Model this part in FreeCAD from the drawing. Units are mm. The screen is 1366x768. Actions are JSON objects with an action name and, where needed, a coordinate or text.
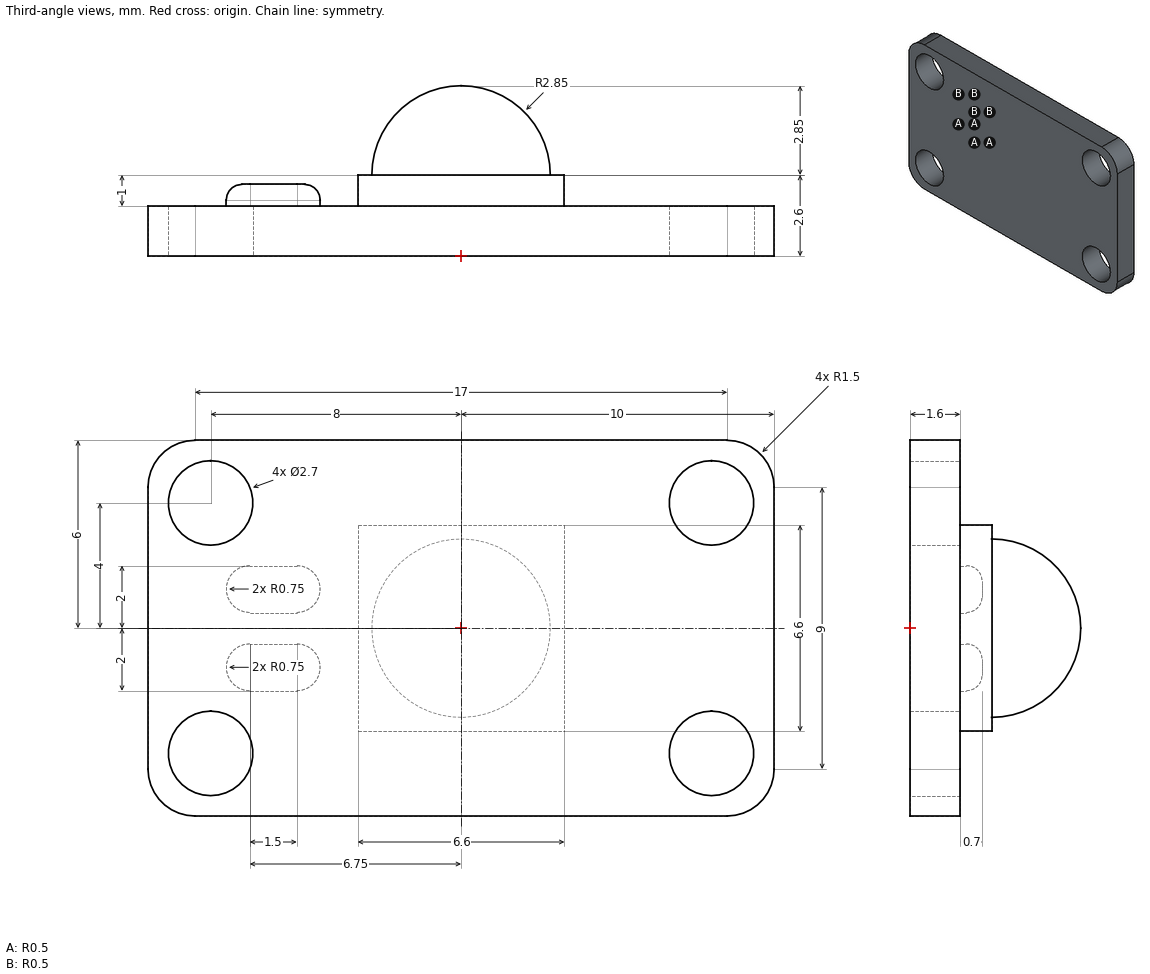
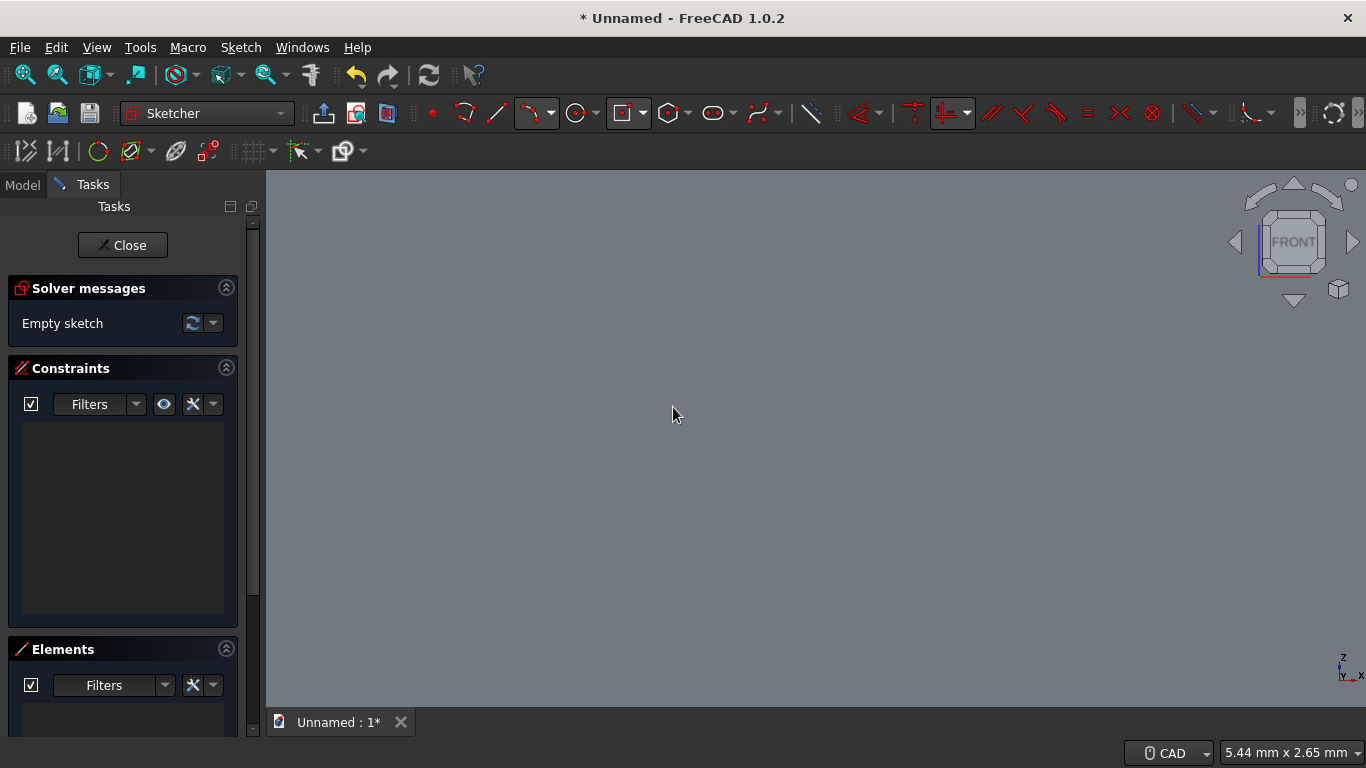
{"action": "left_click", "coordinate": [714, 114]}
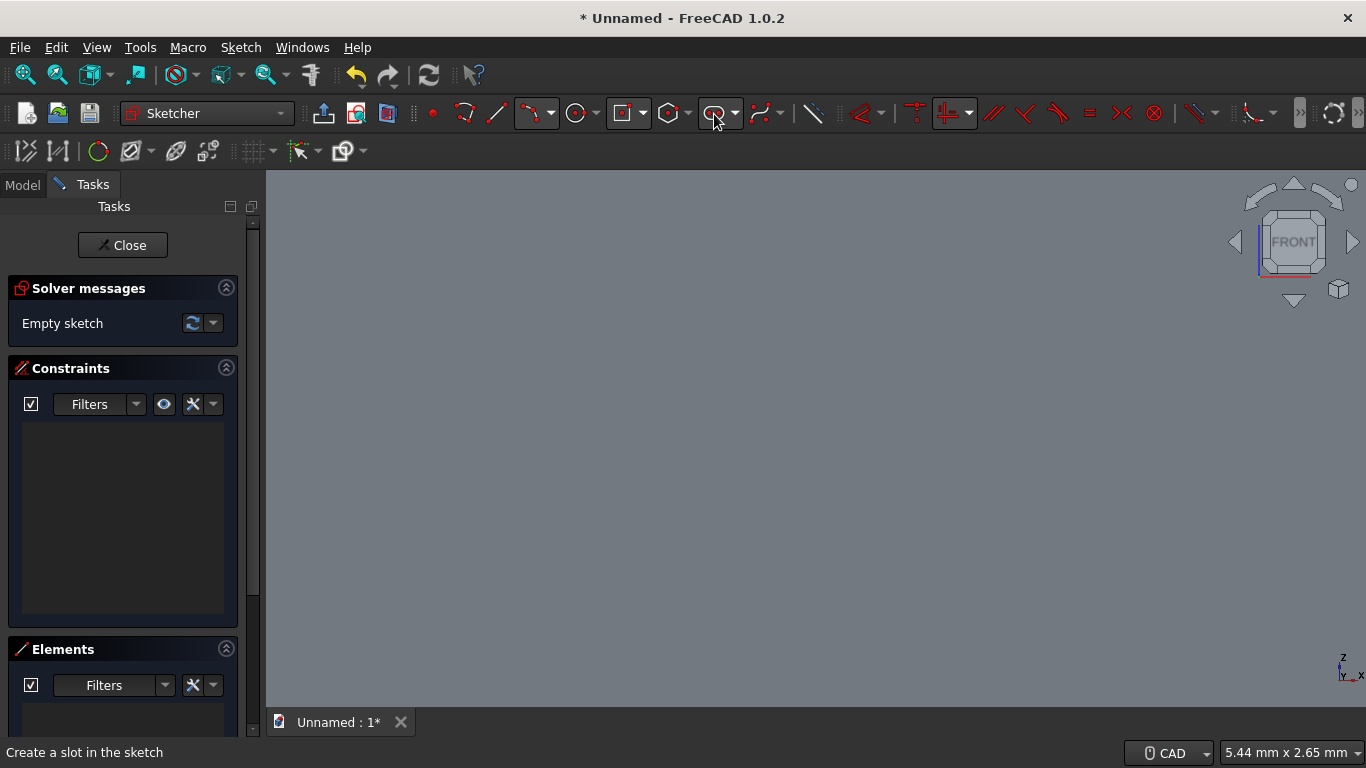
{"action": "left_click", "coordinate": [595, 435]}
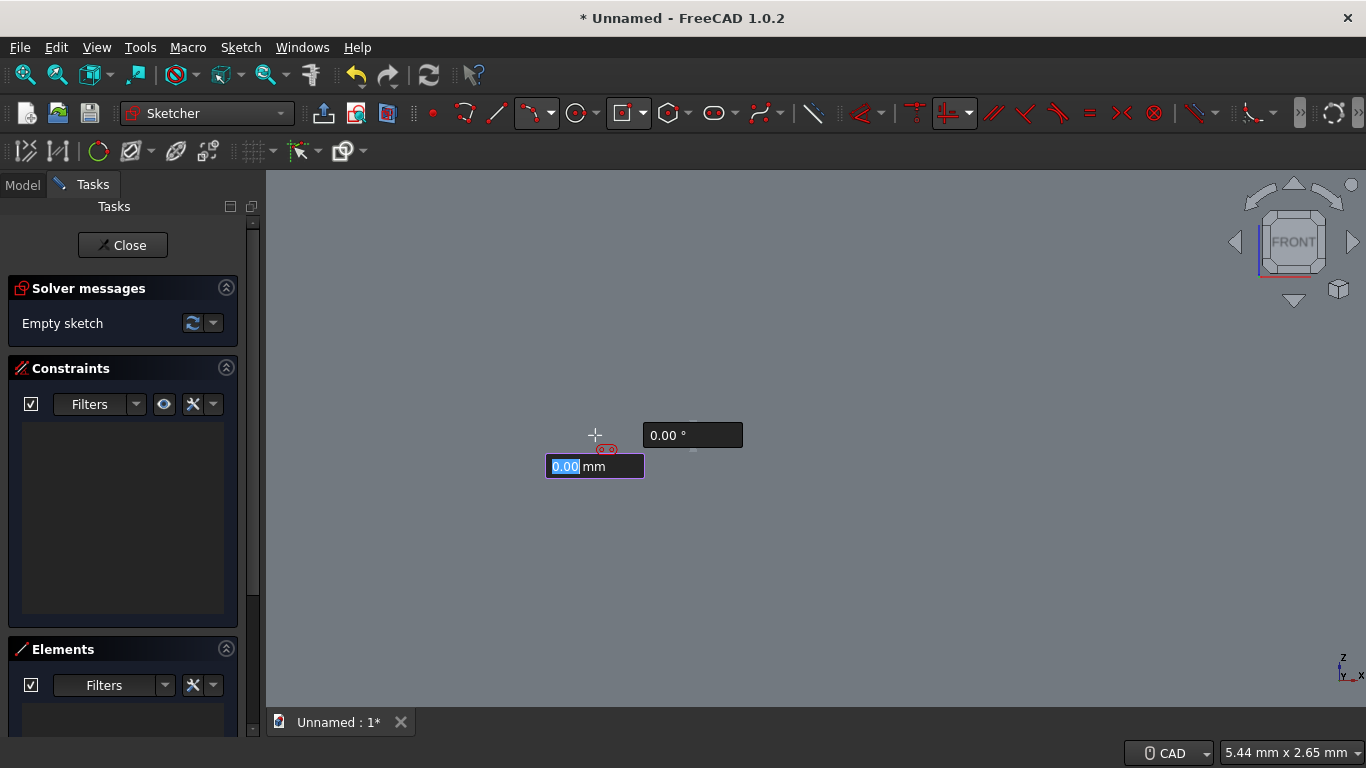
{"action": "left_click", "coordinate": [898, 435]}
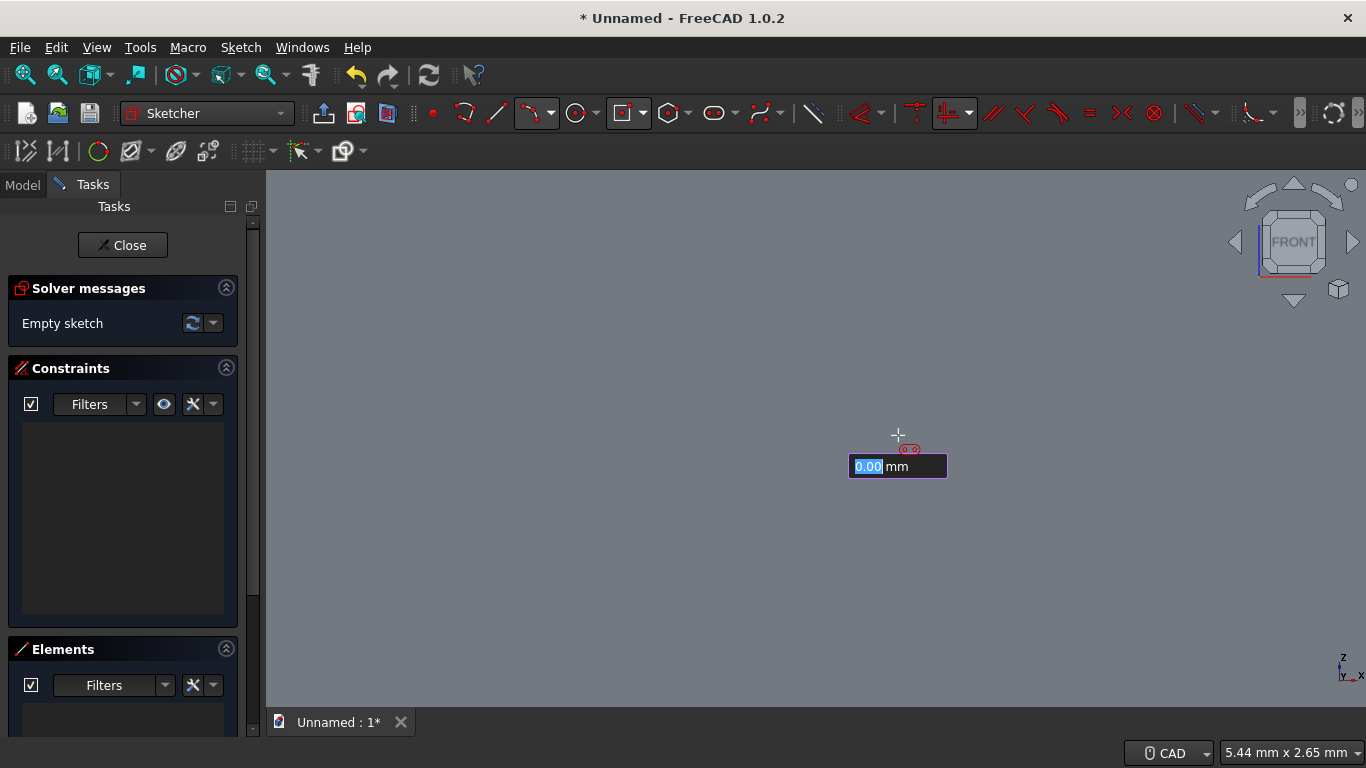
{"action": "left_click", "coordinate": [747, 587]}
{"action": "key", "text": "Escape"}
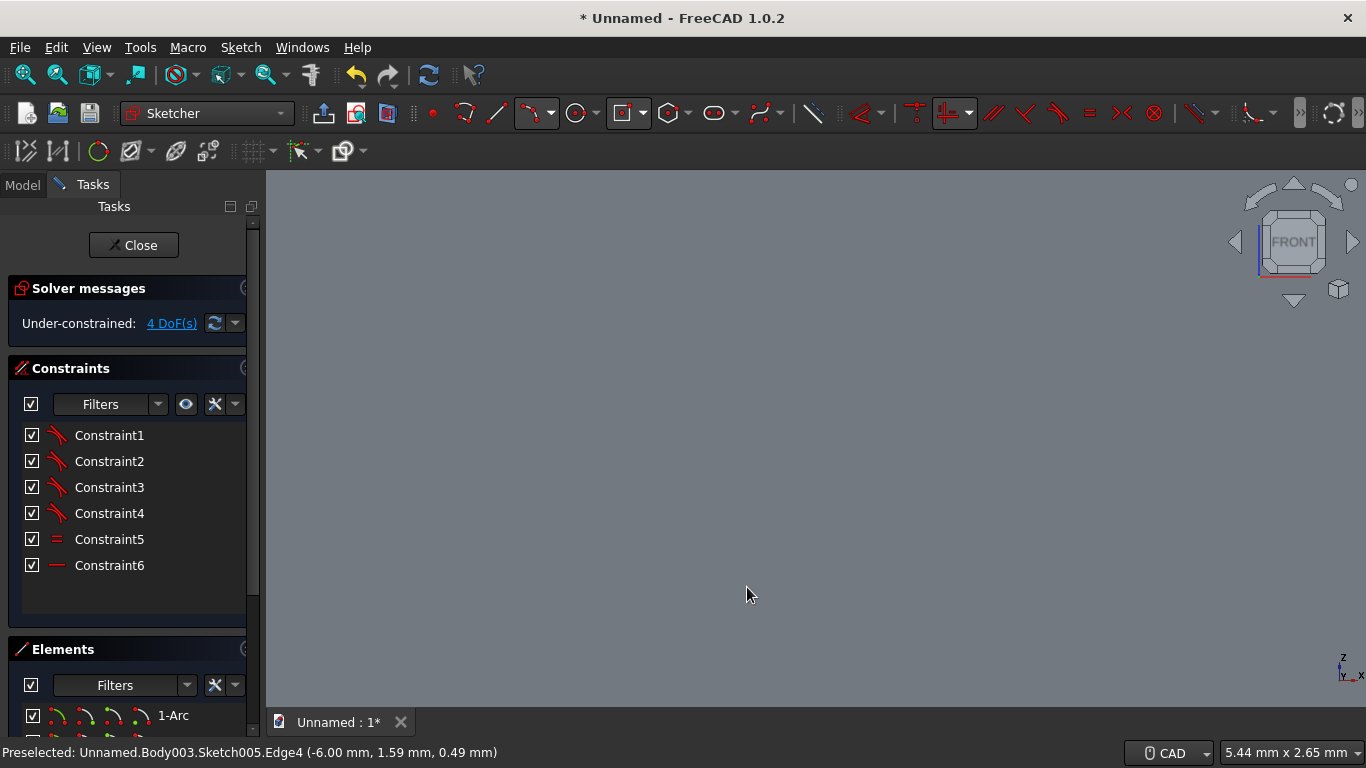
{"action": "left_click", "coordinate": [860, 114]}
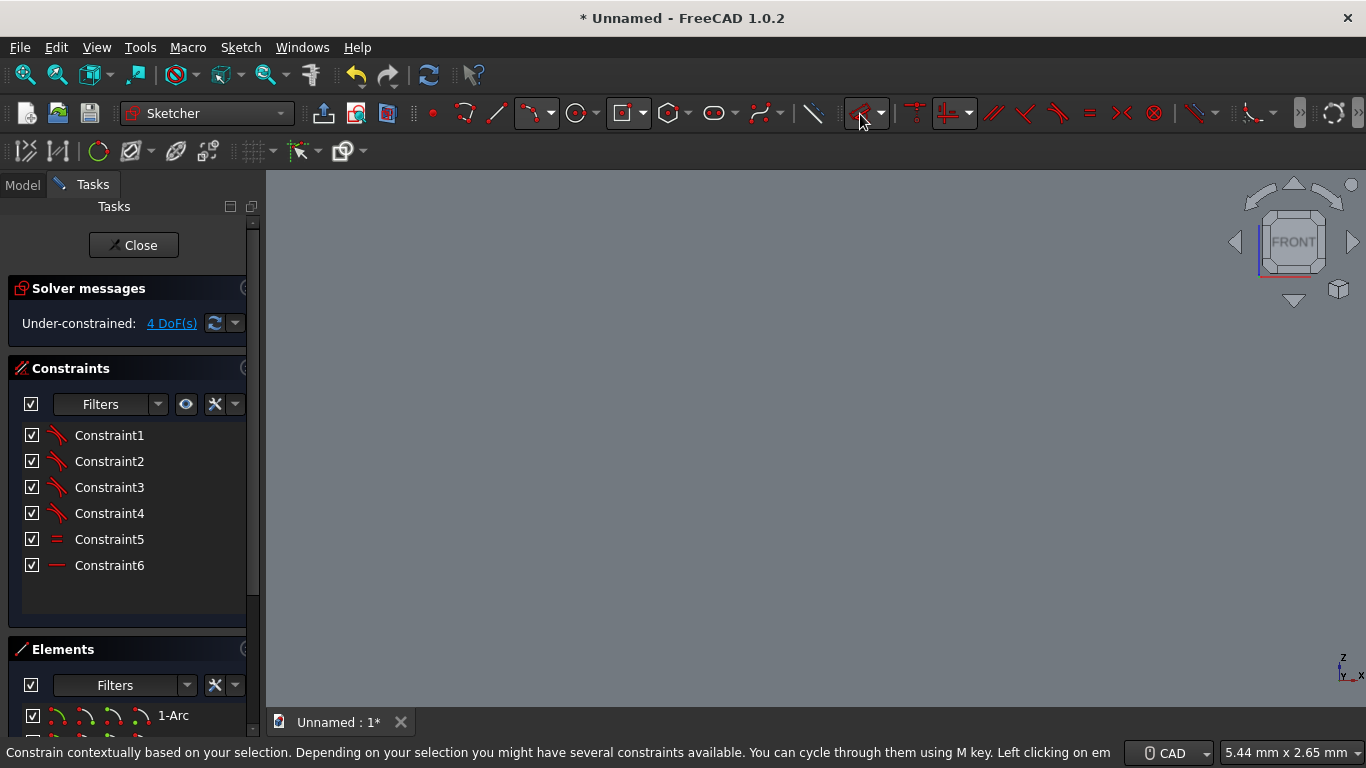
{"action": "left_click", "coordinate": [472, 347]}
{"action": "left_click", "coordinate": [446, 328]}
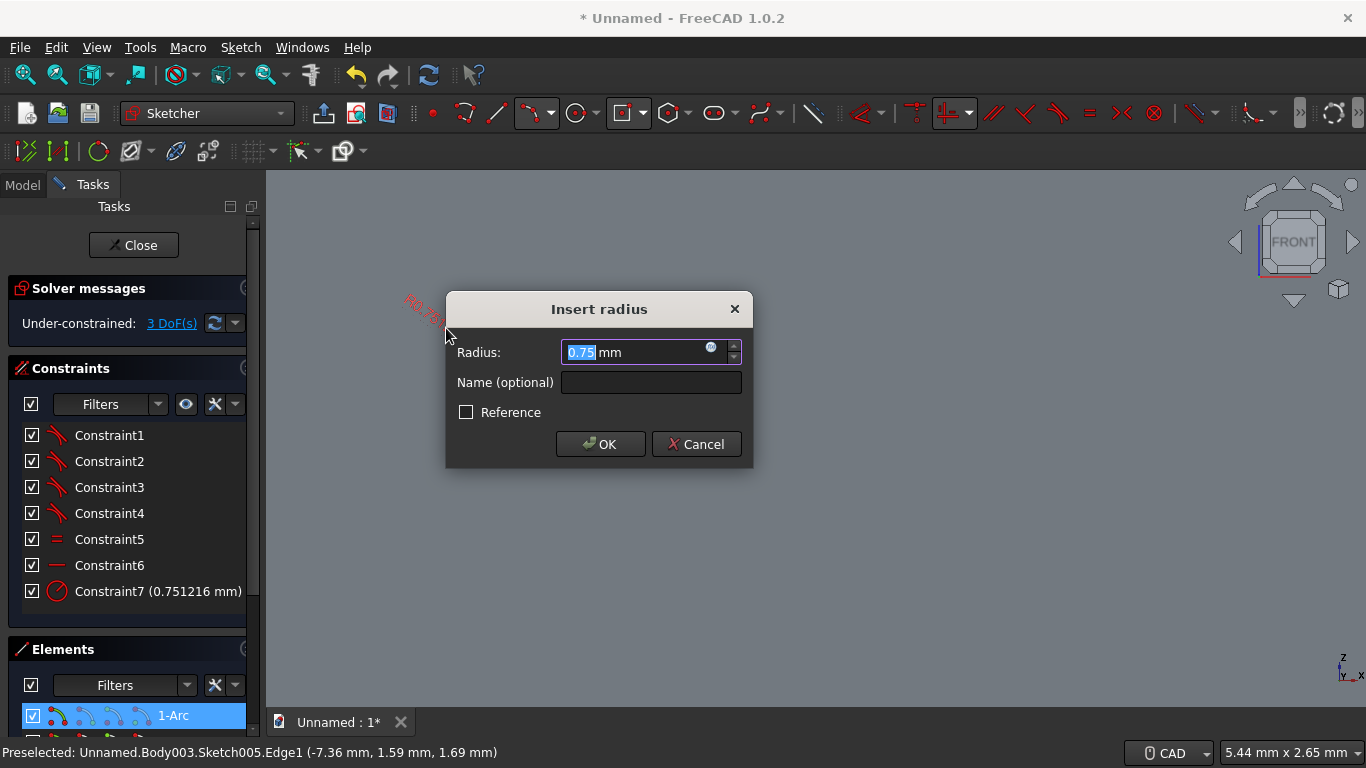
{"action": "type", "text": "0.75"}
{"action": "key", "text": "Return"}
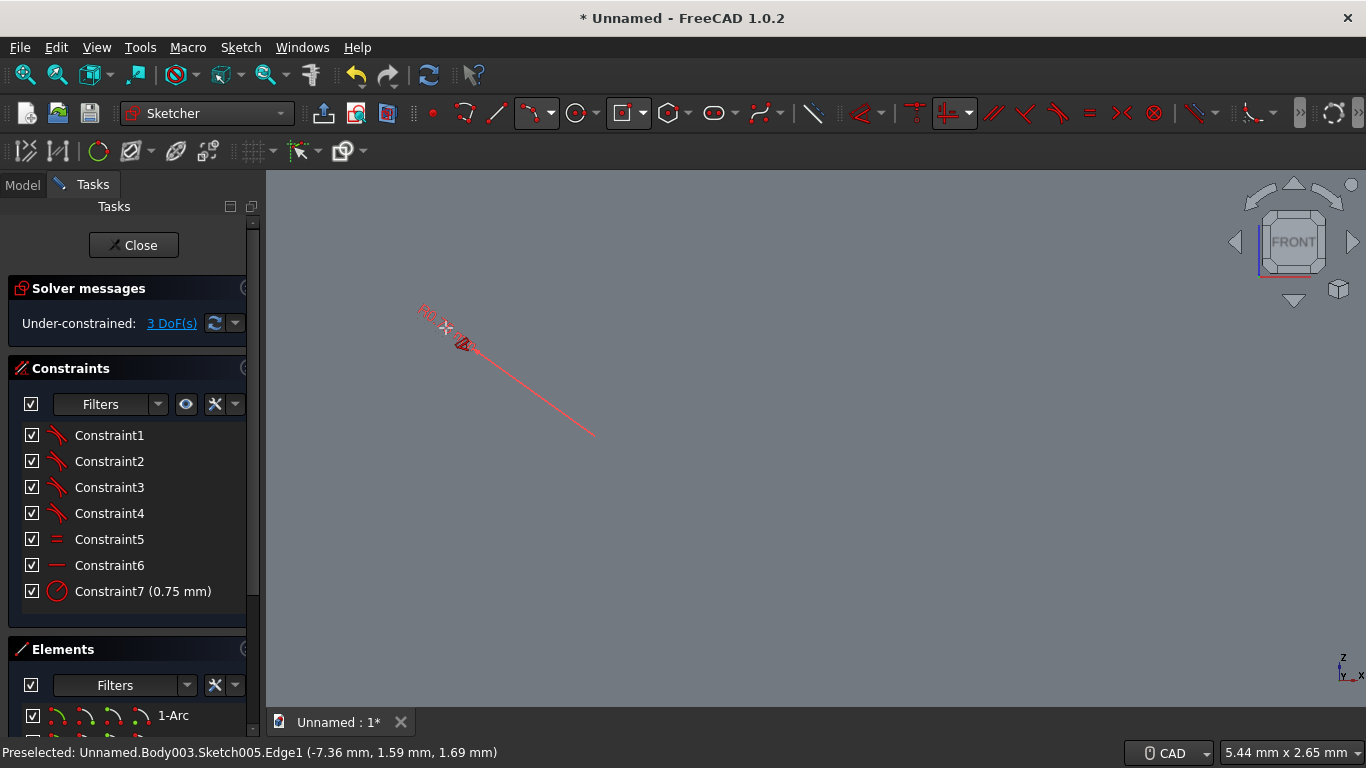
{"action": "left_click", "coordinate": [595, 284]}
{"action": "left_click", "coordinate": [561, 482]}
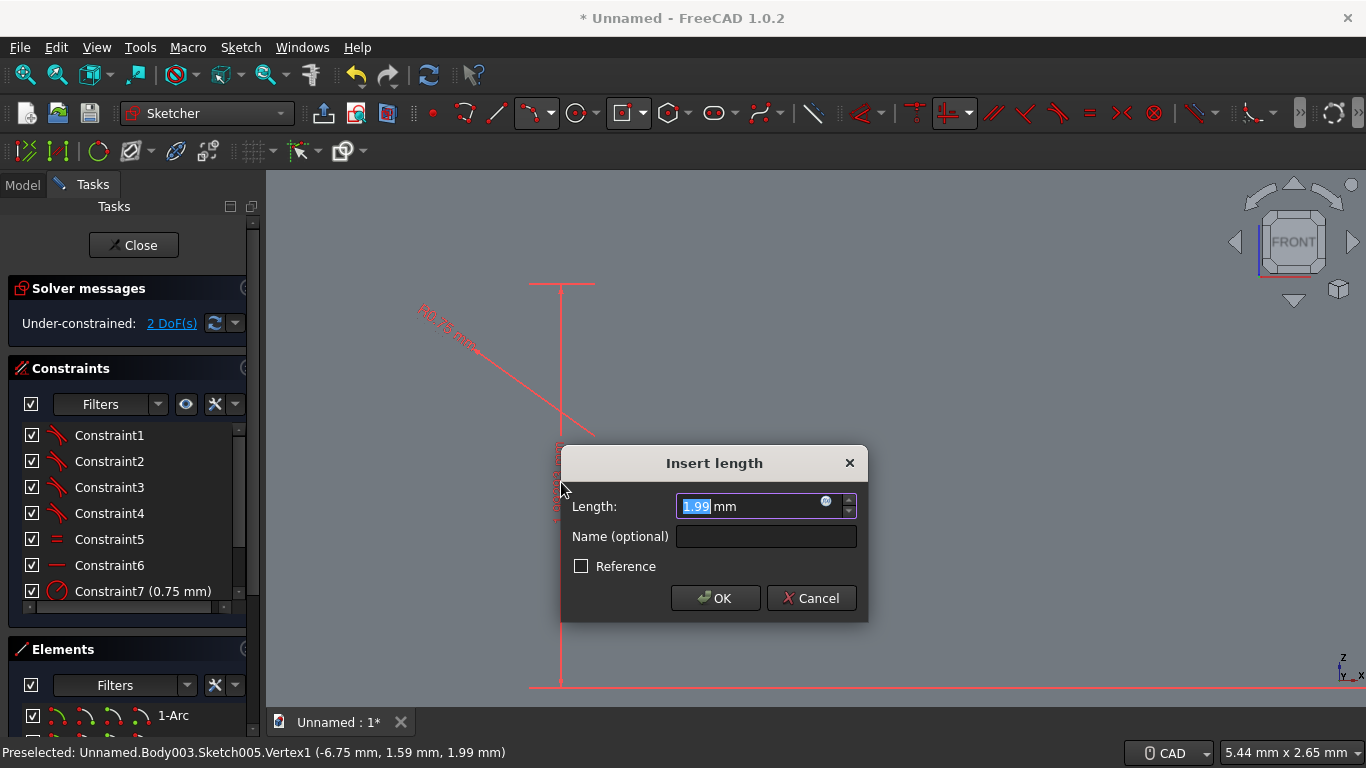
{"action": "type", "text": "2"}
{"action": "key", "text": "Return"}